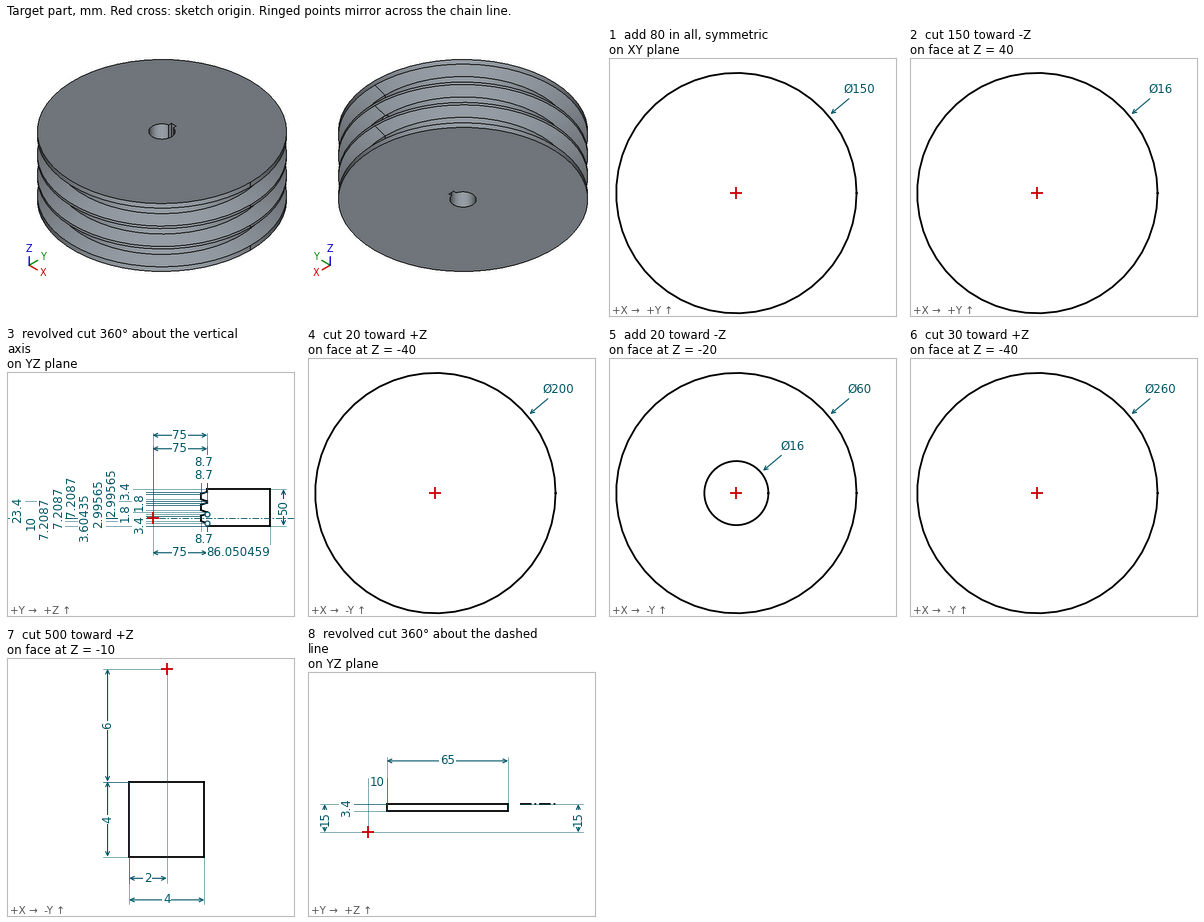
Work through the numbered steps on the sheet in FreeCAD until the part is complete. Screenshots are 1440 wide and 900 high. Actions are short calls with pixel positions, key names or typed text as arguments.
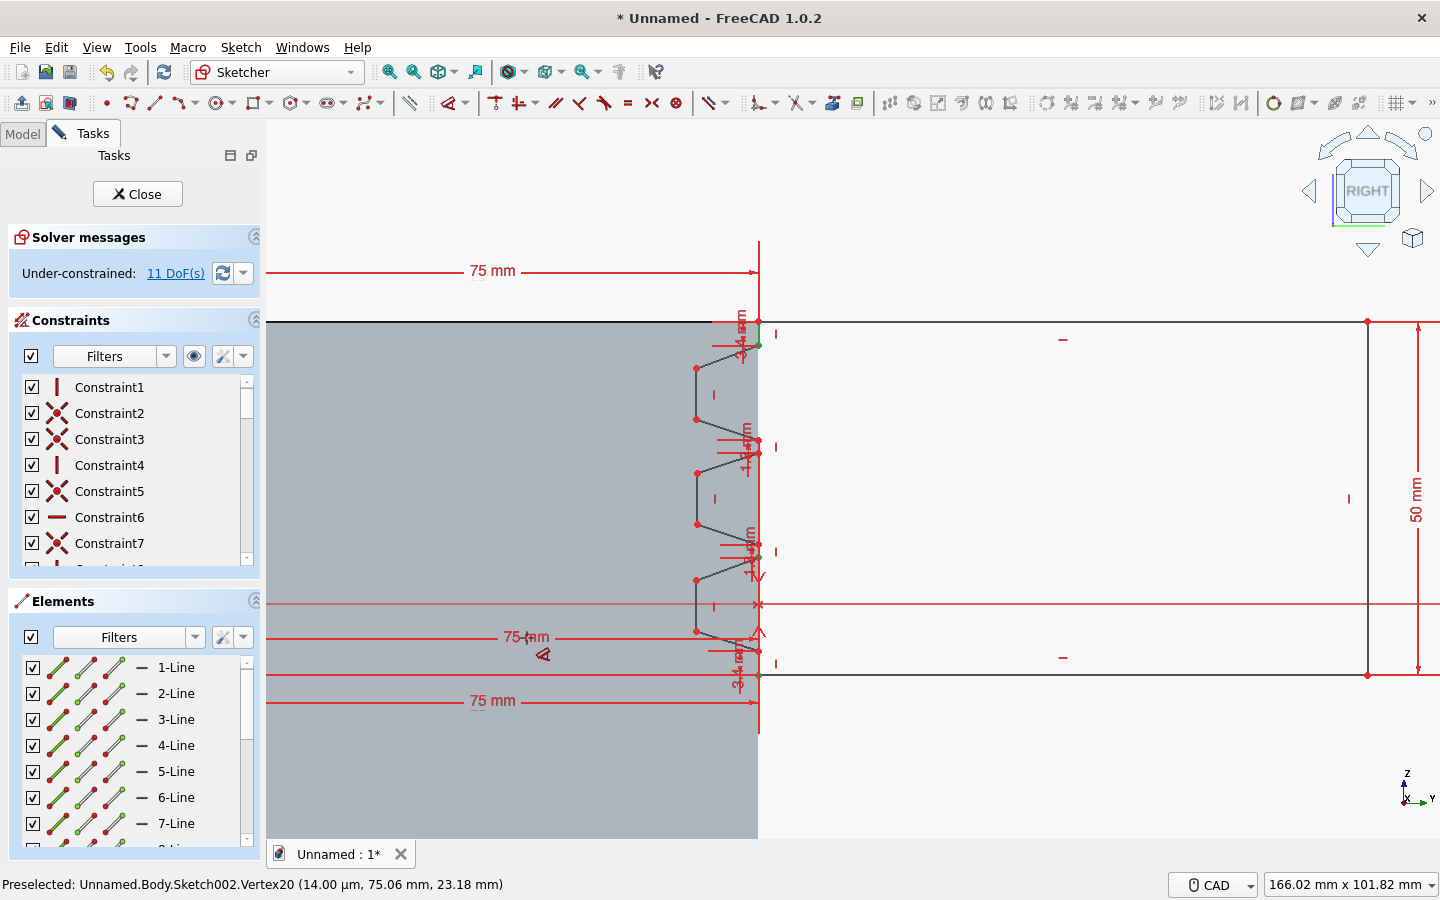
click(715, 637)
click(728, 685)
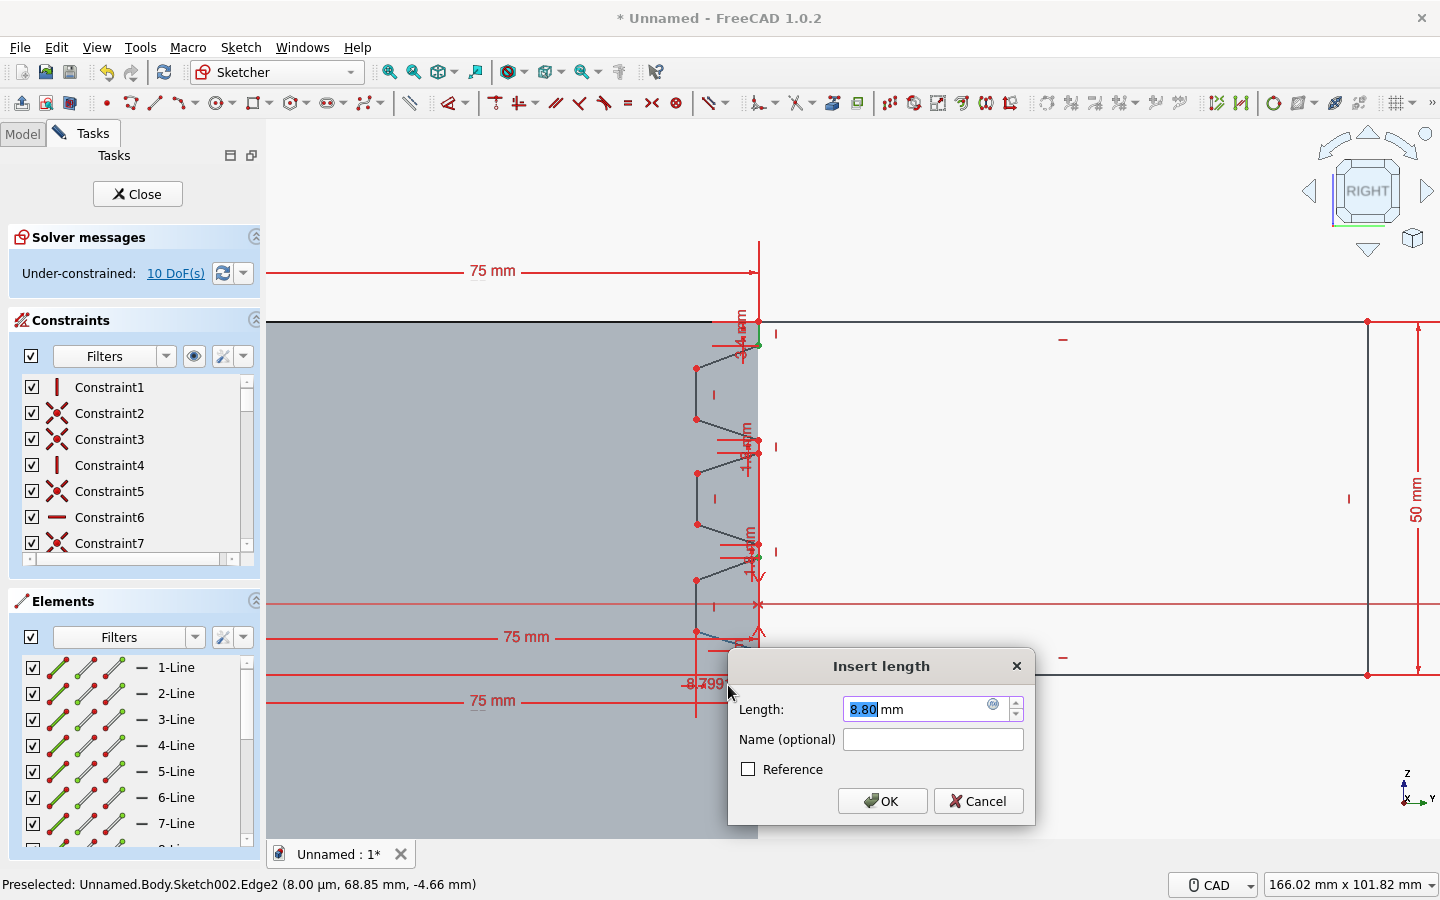
text(8.7)
key(Return)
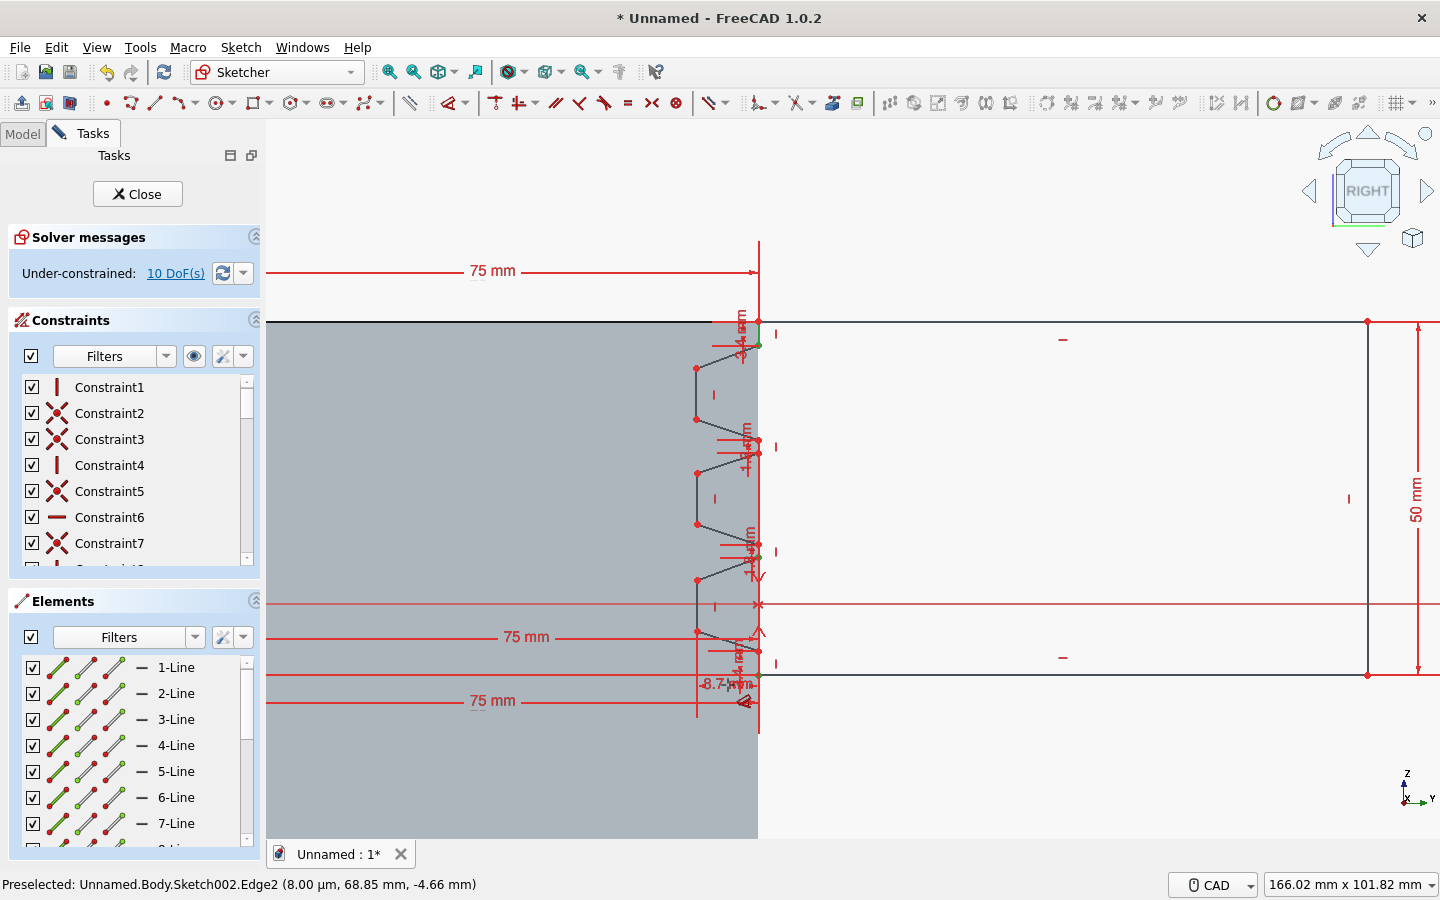
click(740, 353)
click(728, 312)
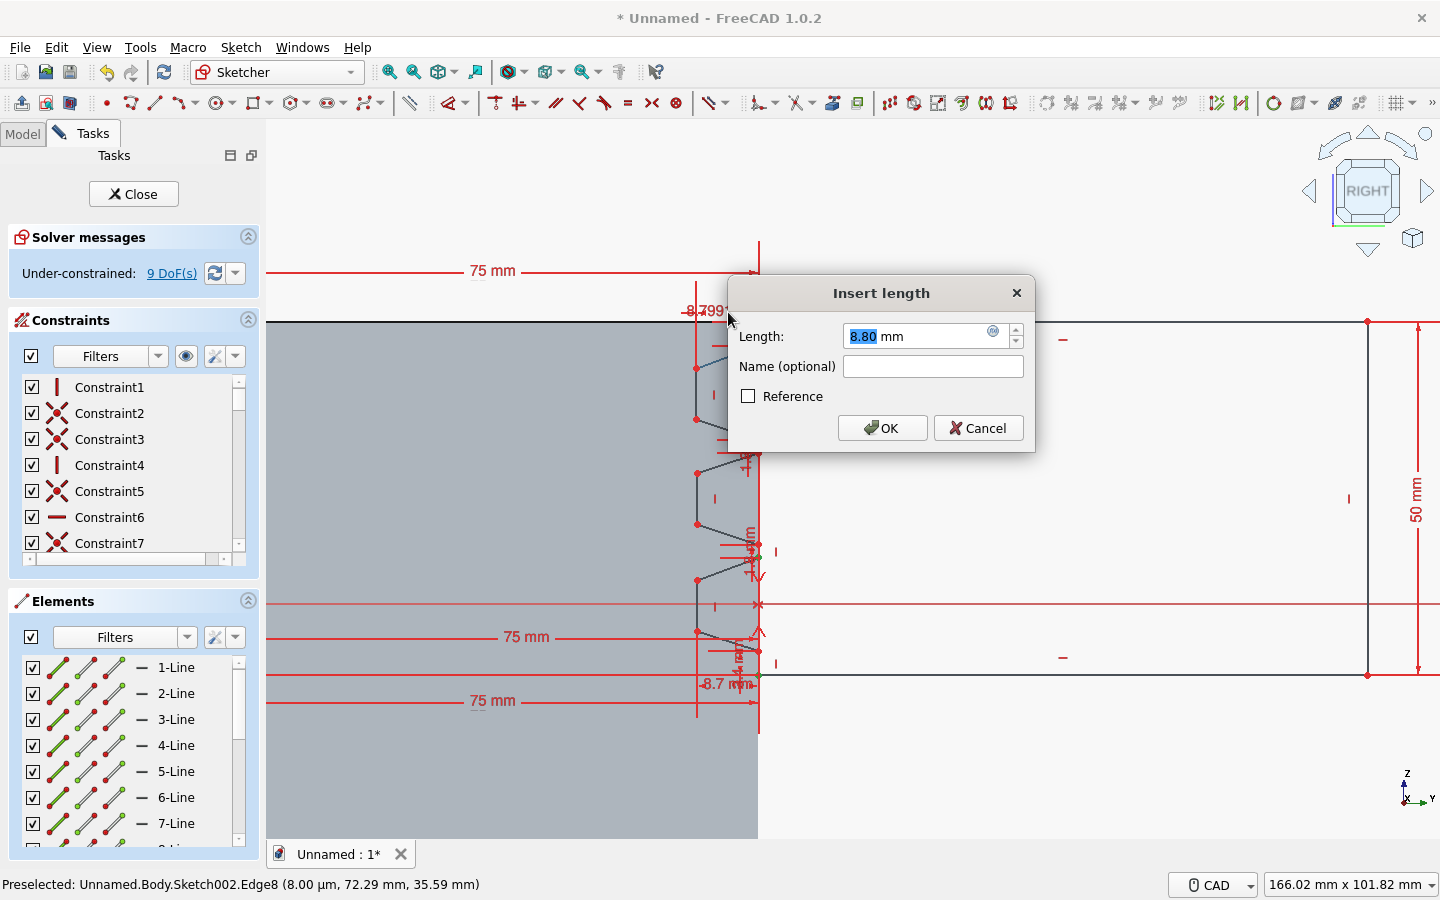
text(8.7)
key(Return)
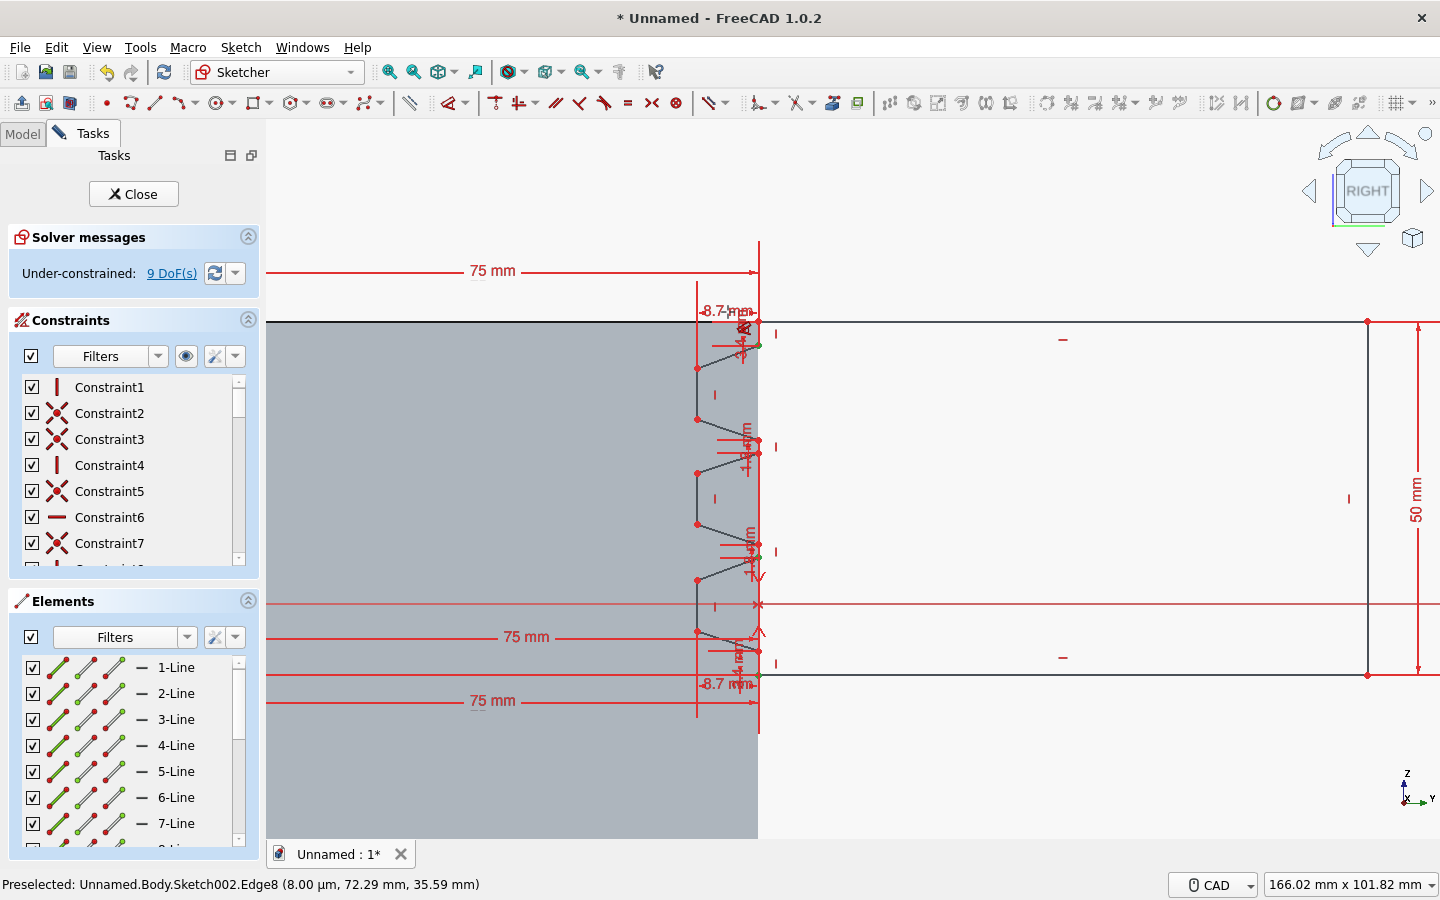
click(740, 459)
click(742, 419)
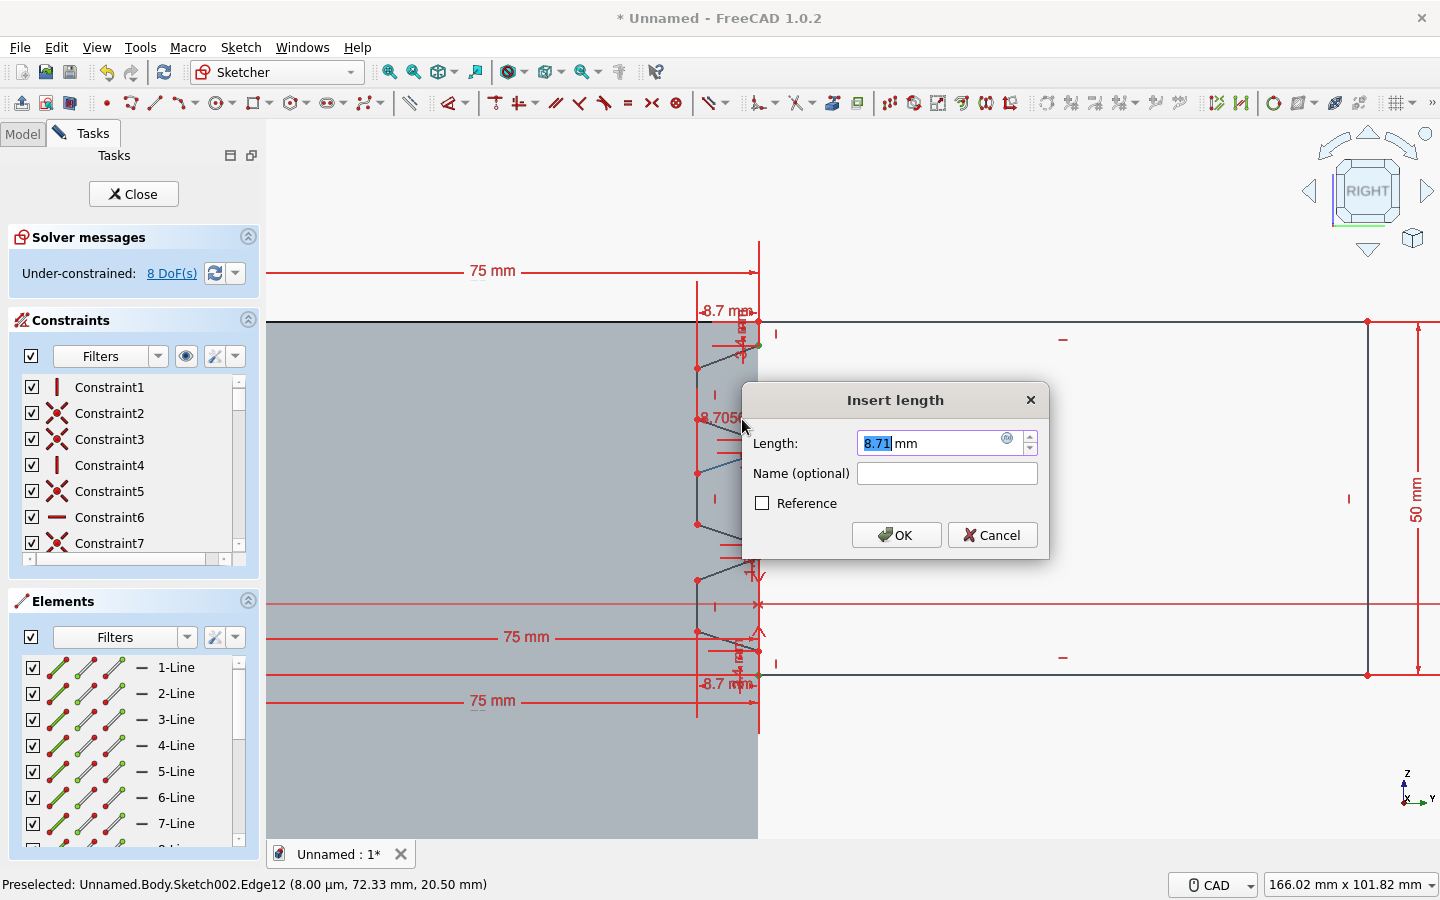
text(8.7)
key(Return)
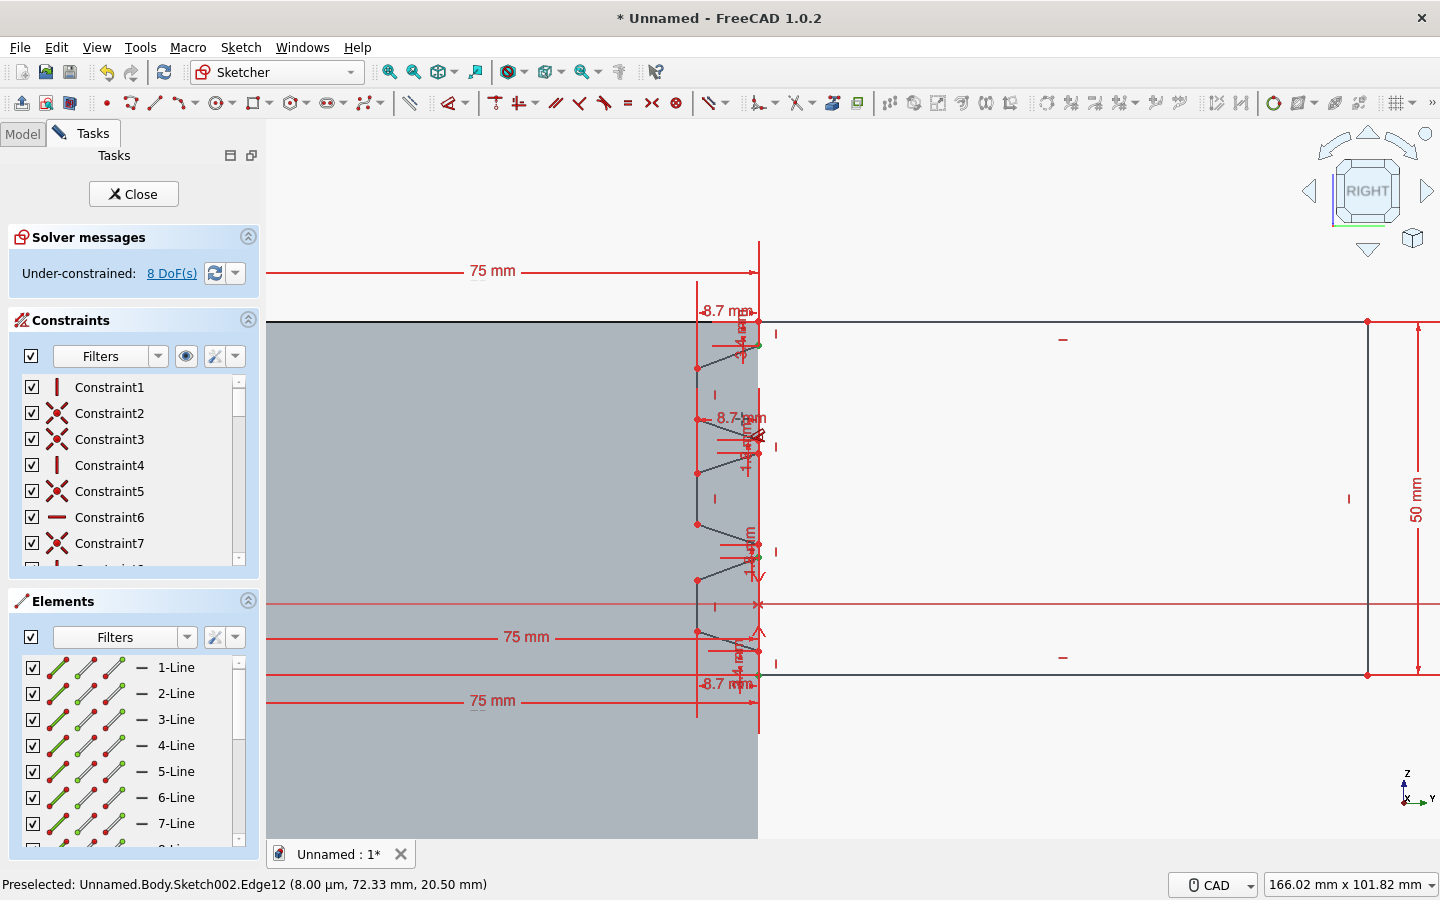
click(759, 440)
click(793, 522)